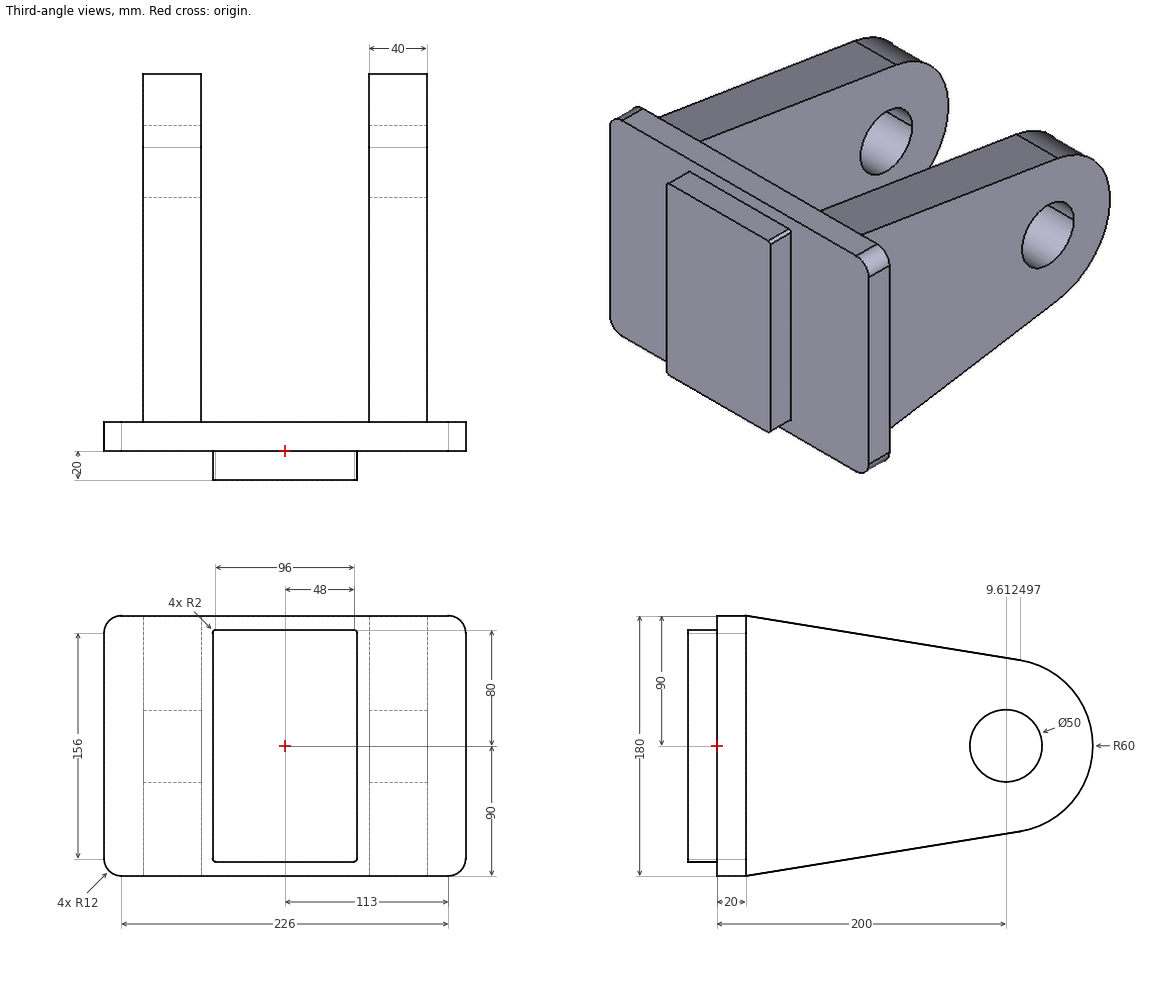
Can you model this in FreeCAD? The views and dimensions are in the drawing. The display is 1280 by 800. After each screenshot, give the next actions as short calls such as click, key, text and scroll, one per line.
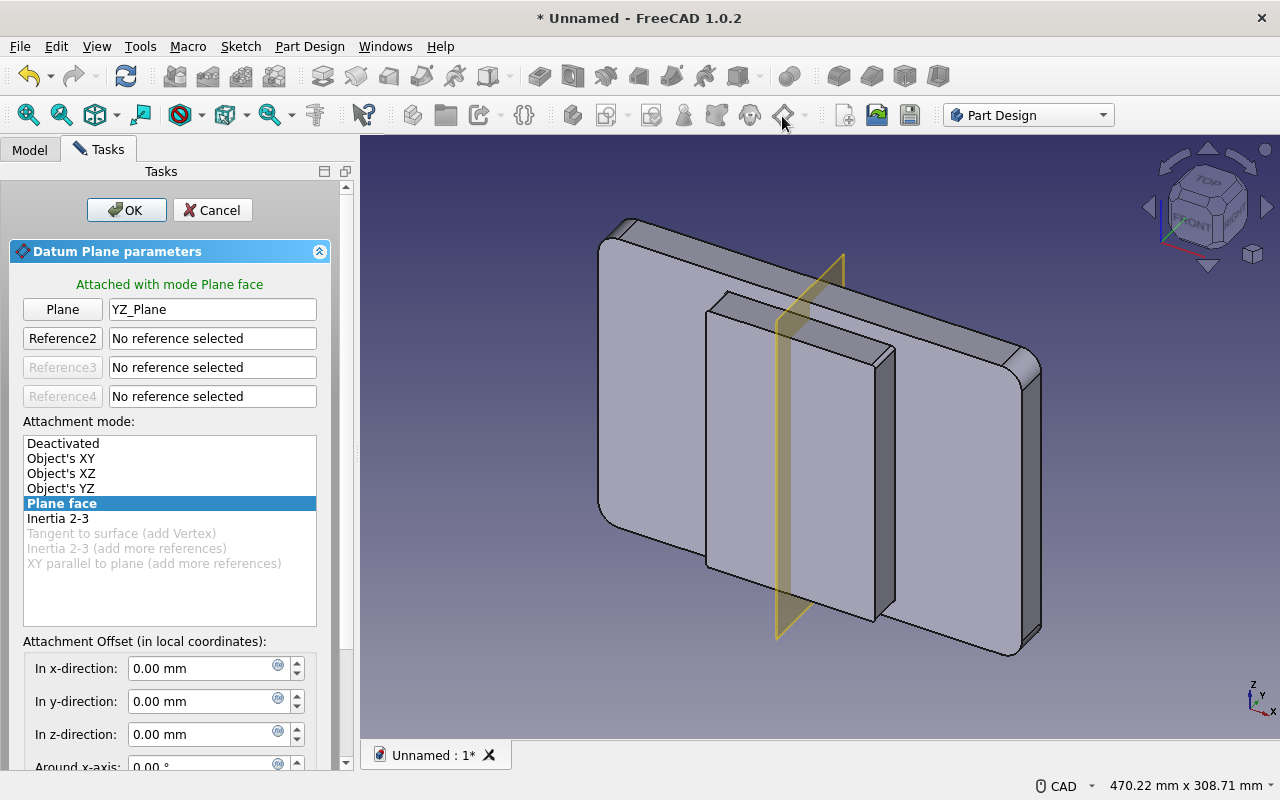
triple_click(210, 734)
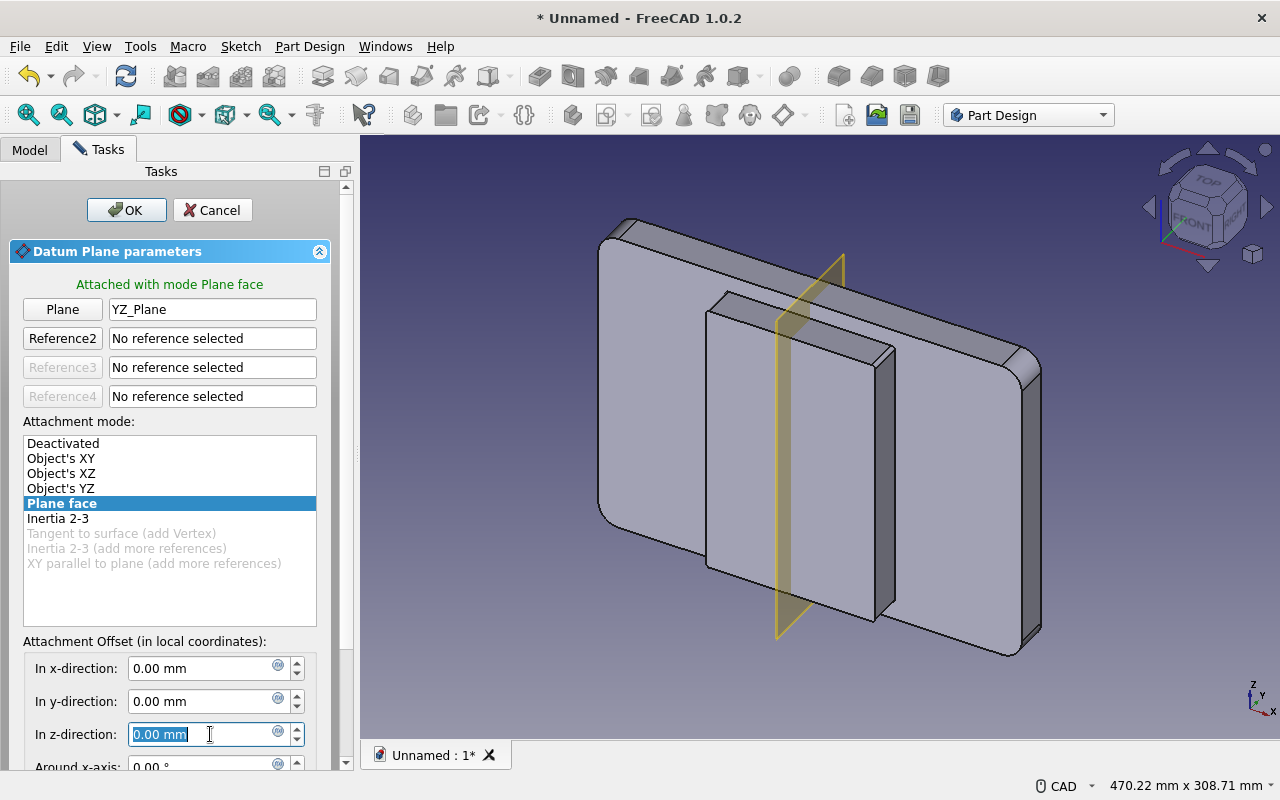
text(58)
key(Tab)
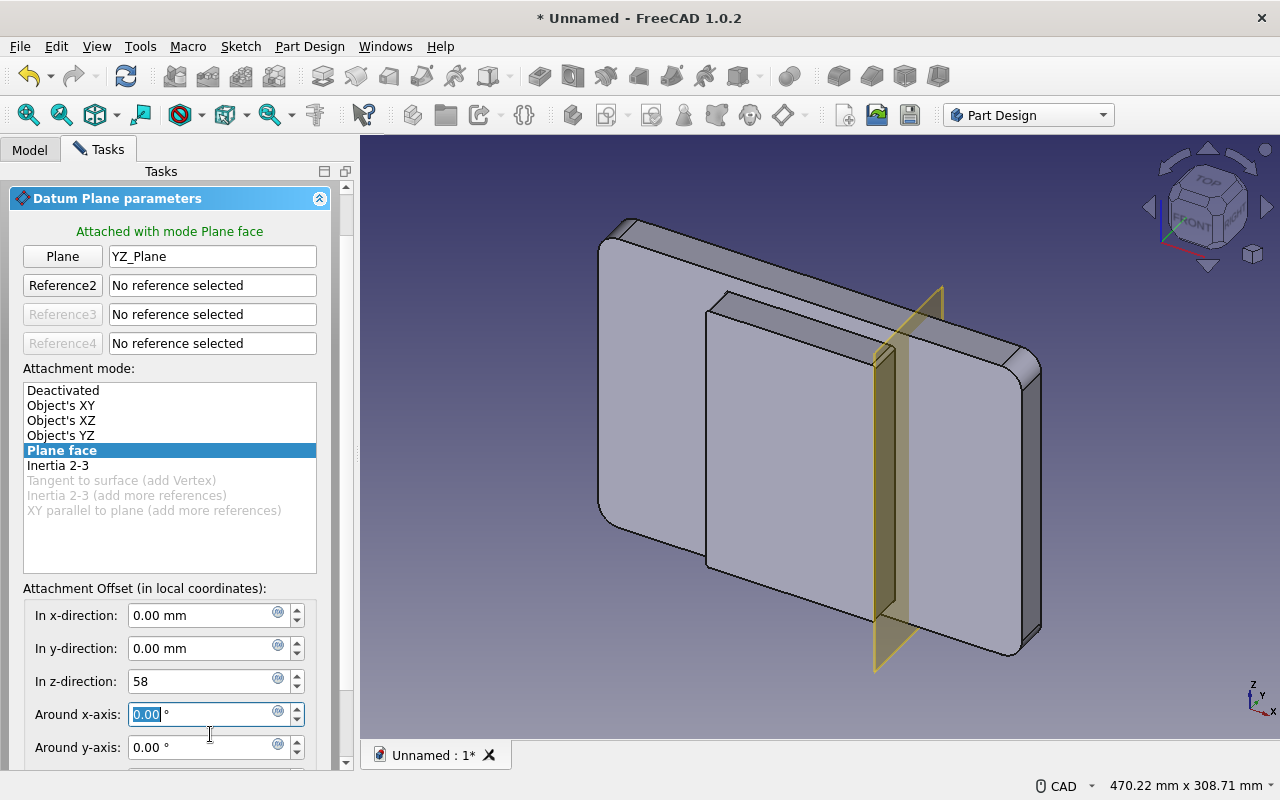
scroll(346, 476, up, 2)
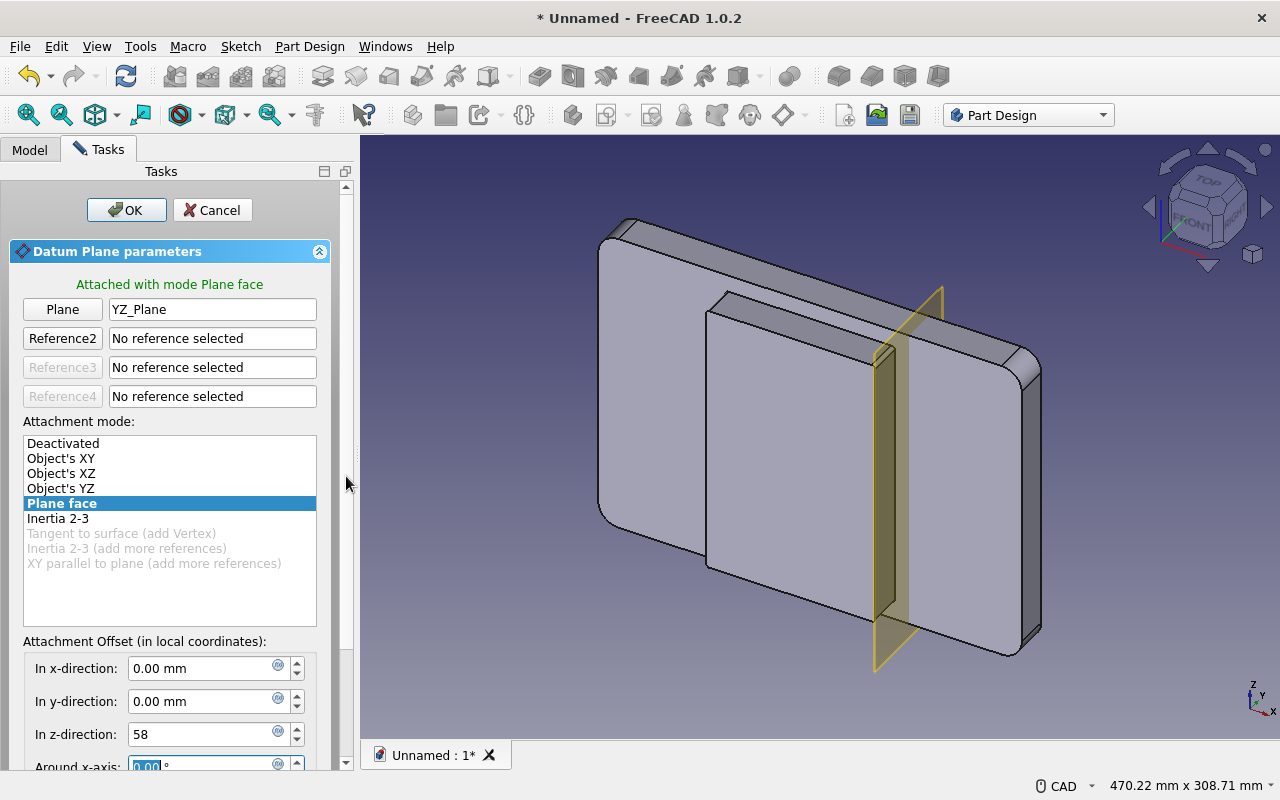
click(127, 210)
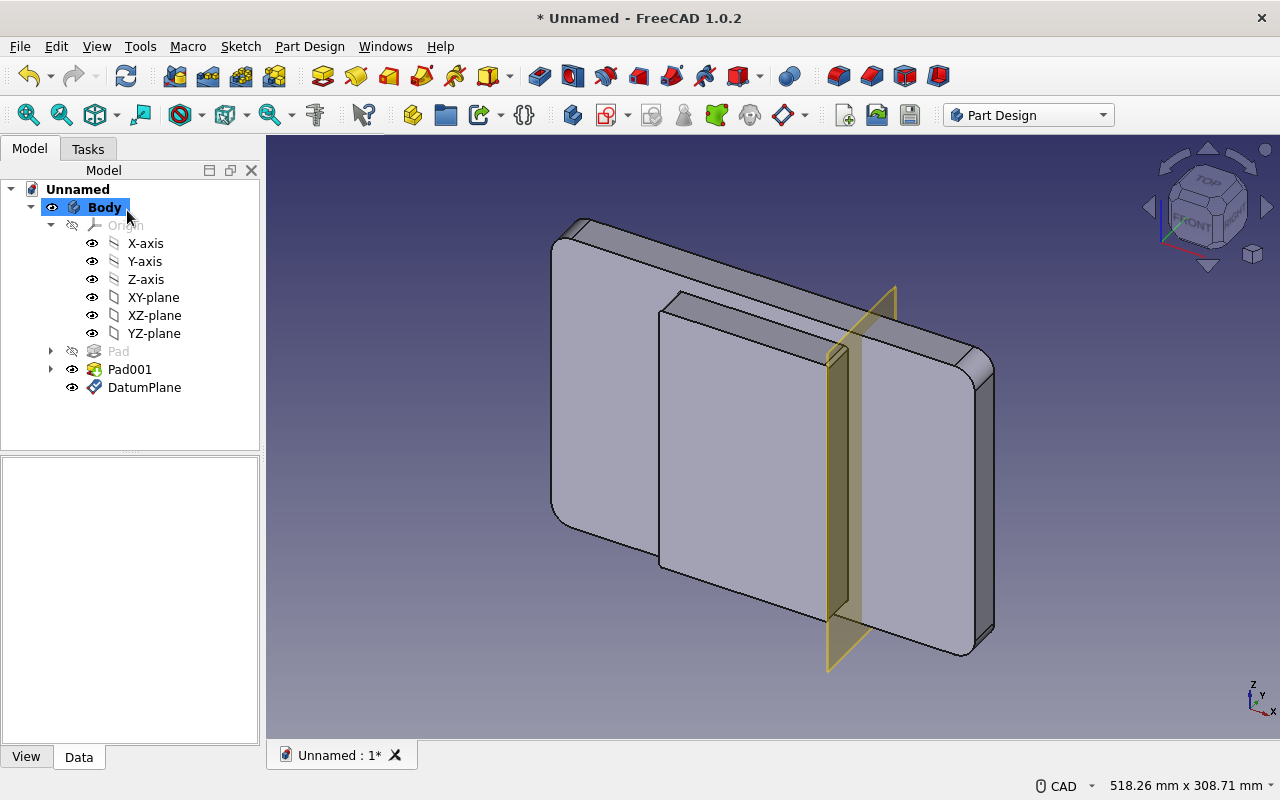
click(117, 387)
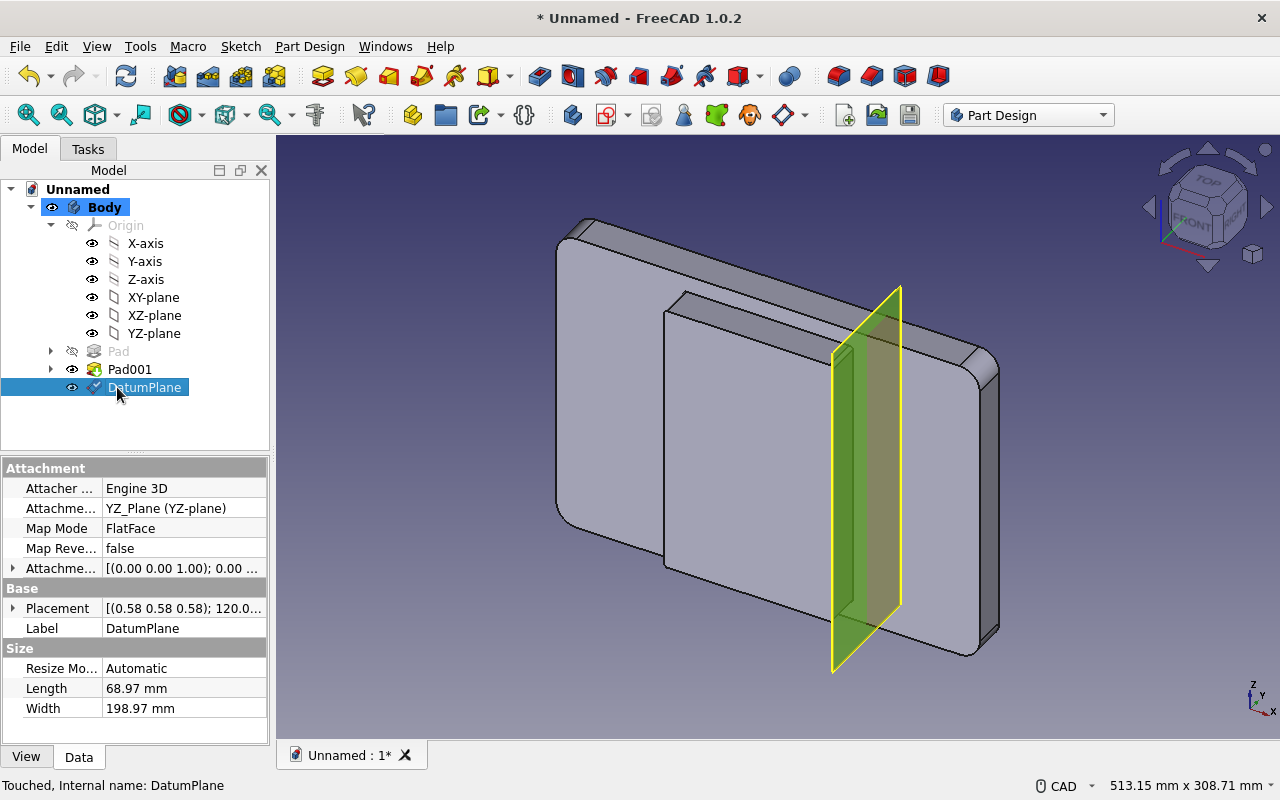
click(606, 116)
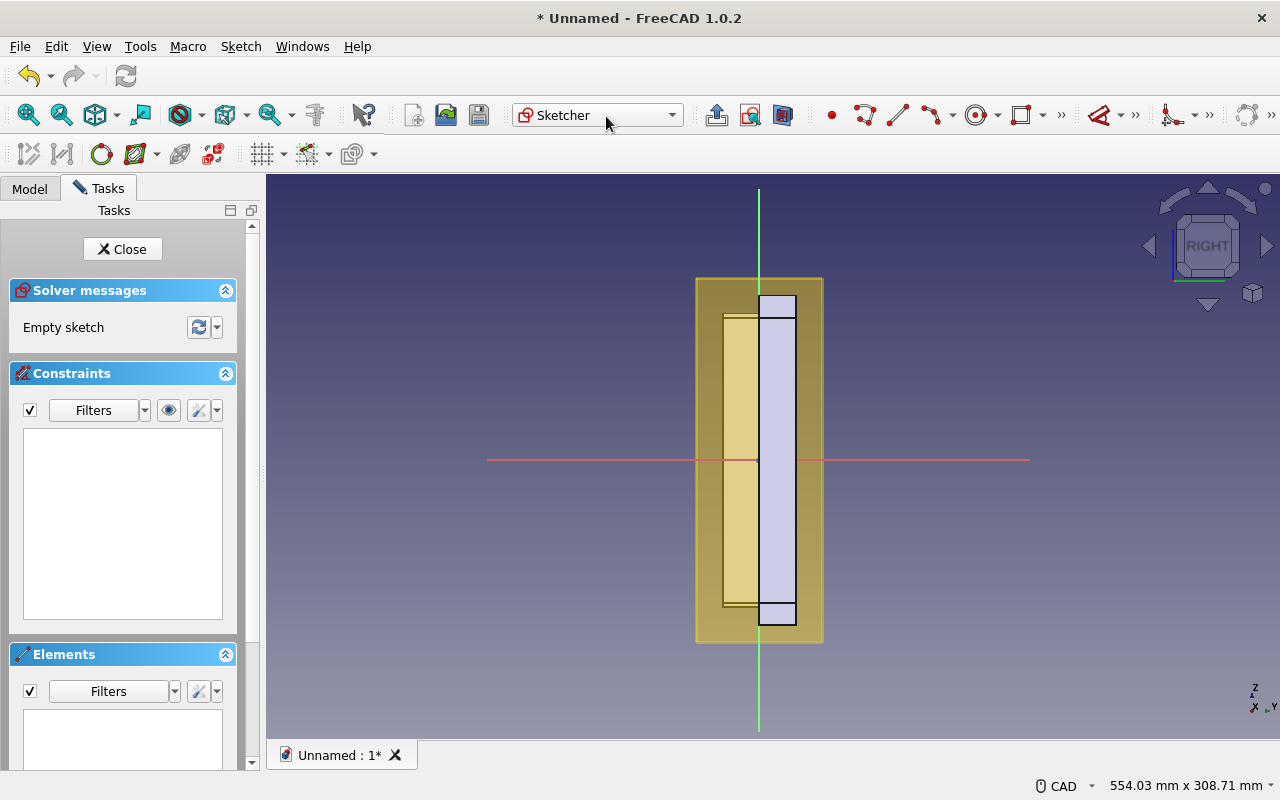
click(783, 116)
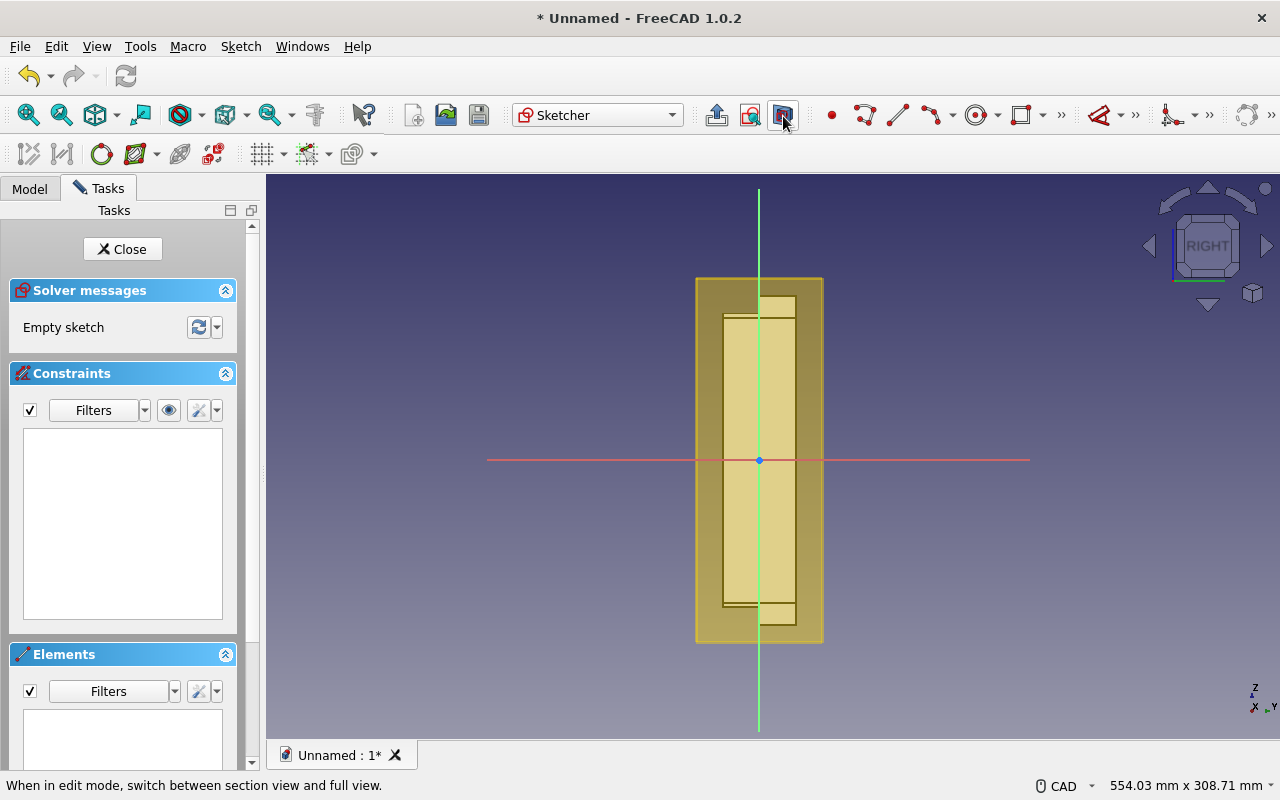
scroll(294, 439, down, 1)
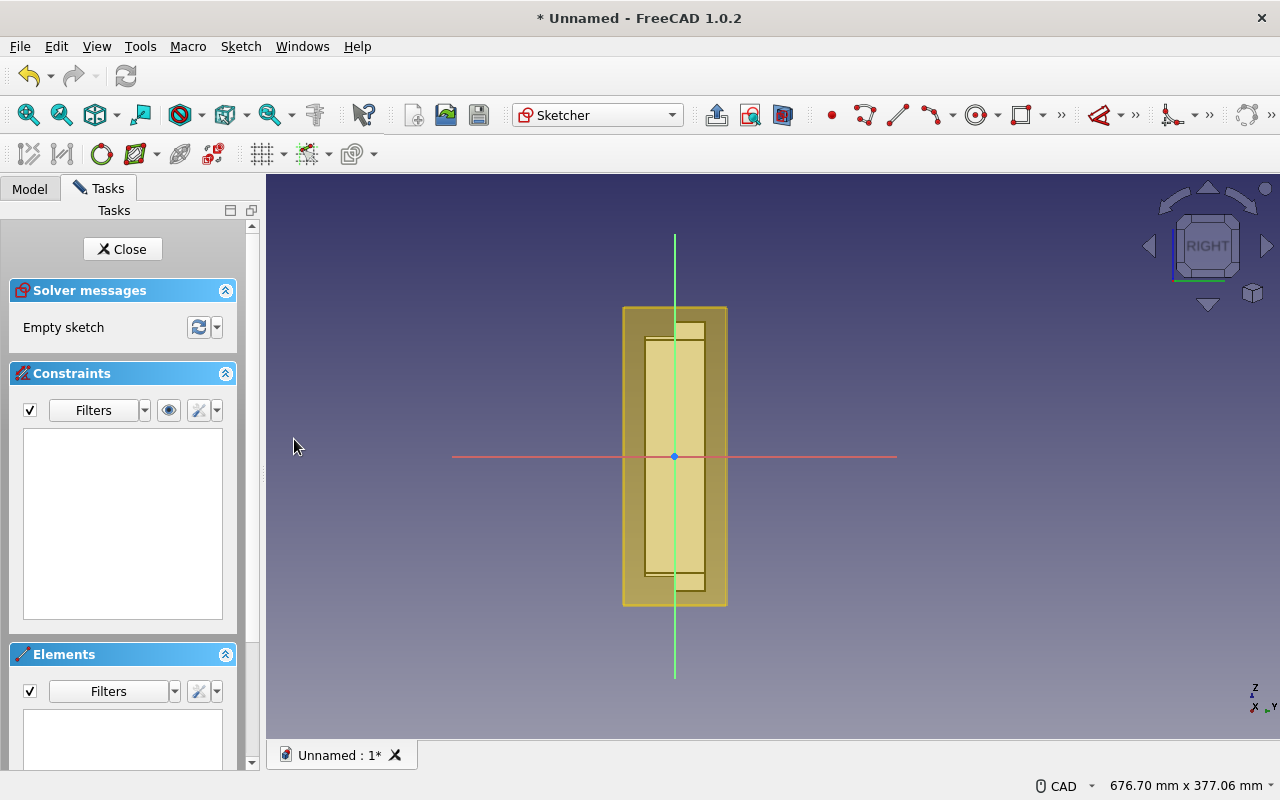
click(865, 116)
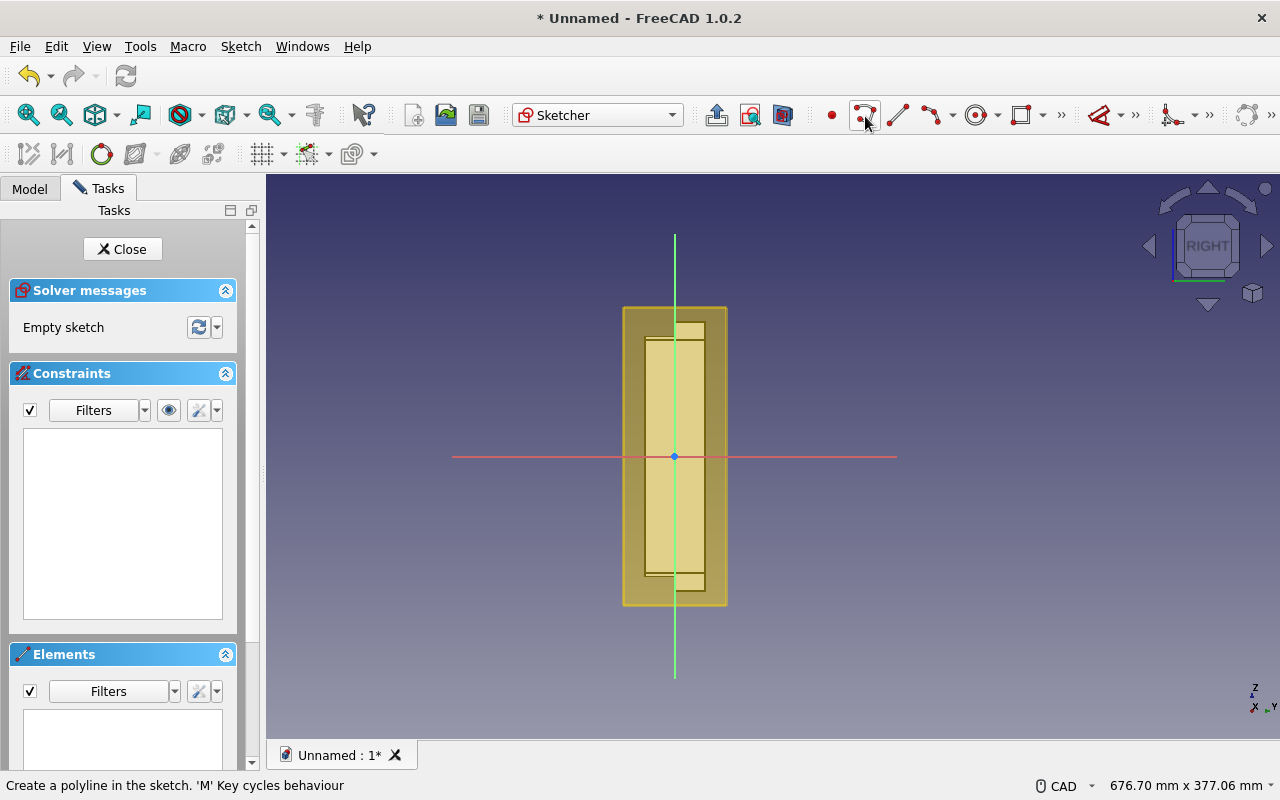
click(989, 368)
click(705, 322)
click(705, 591)
click(989, 545)
right_click(989, 545)